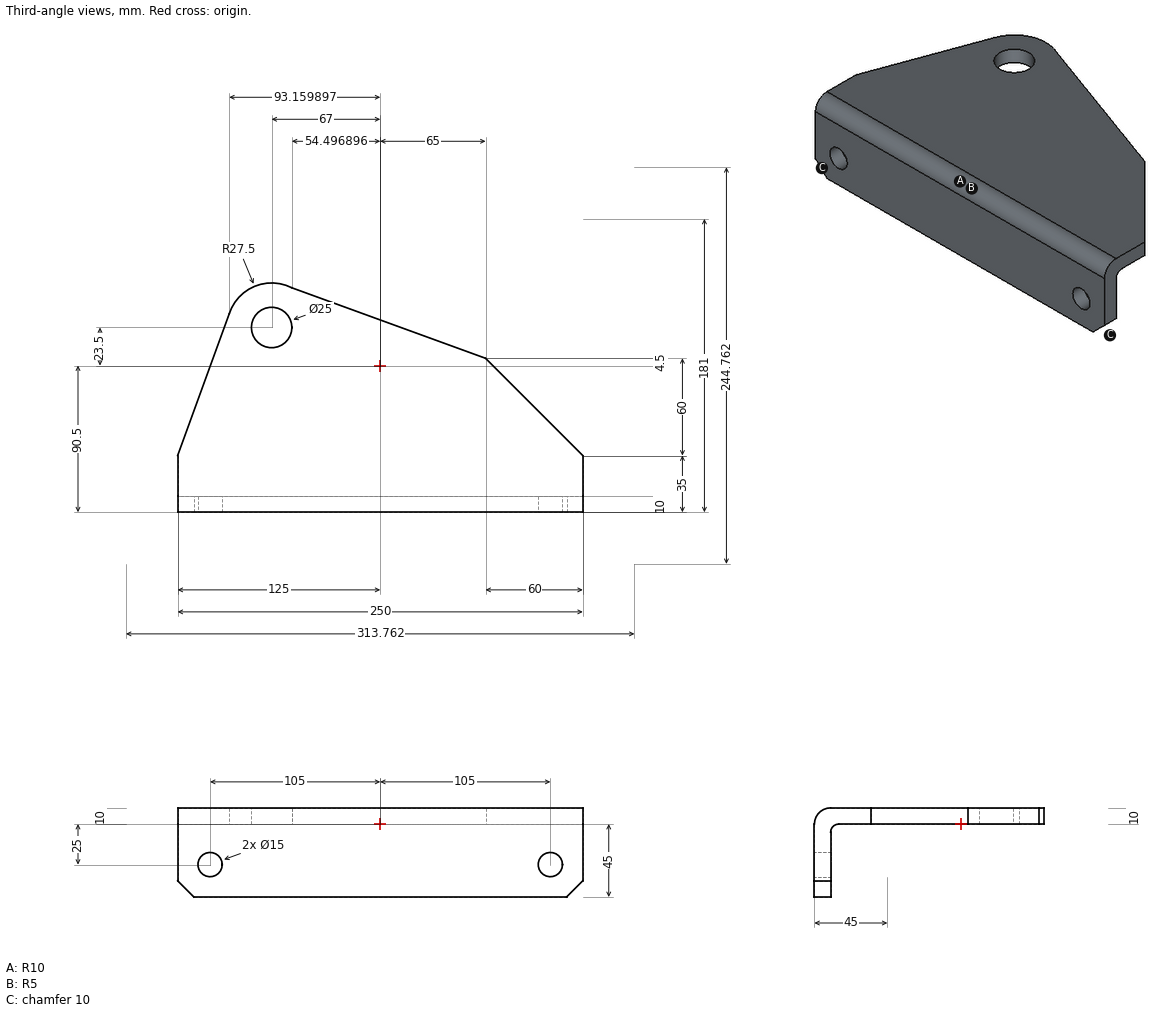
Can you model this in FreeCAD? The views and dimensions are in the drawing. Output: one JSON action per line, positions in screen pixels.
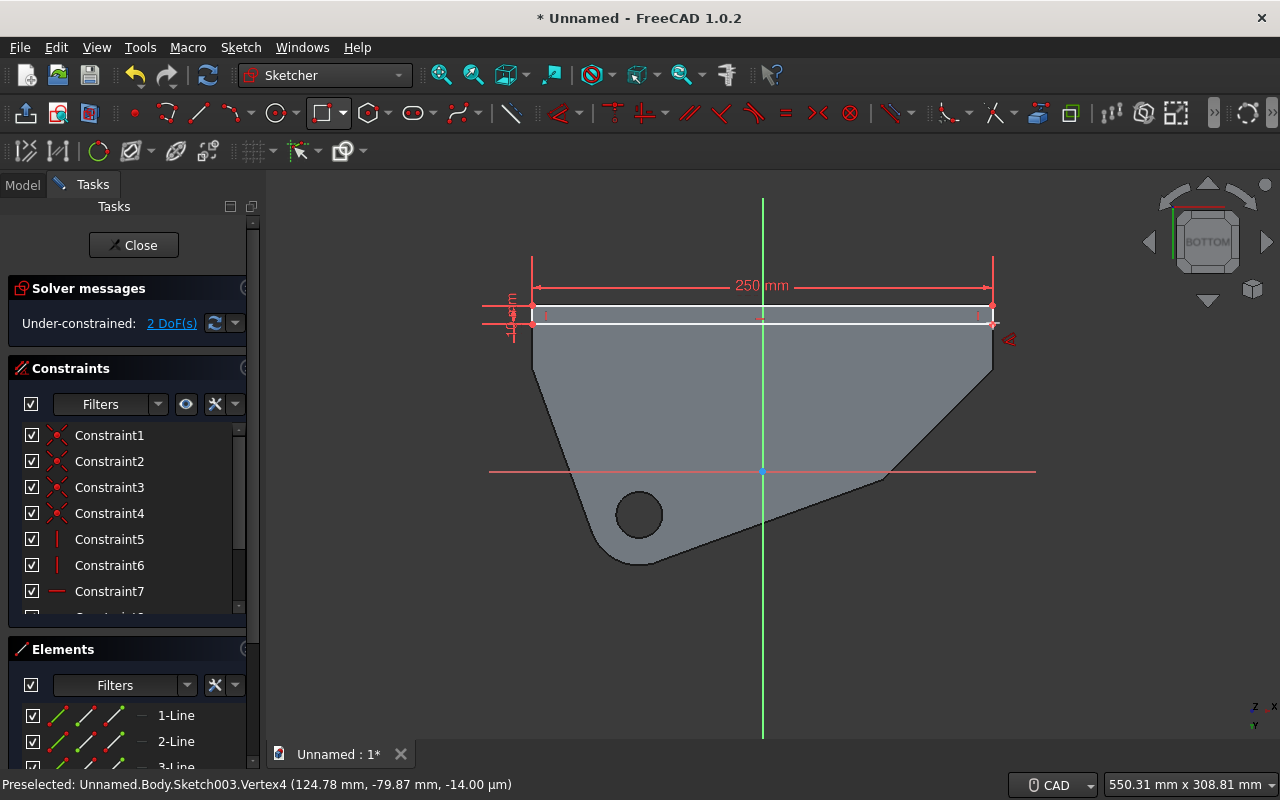
{"action": "left_click", "coordinate": [532, 306]}
{"action": "left_click", "coordinate": [647, 506]}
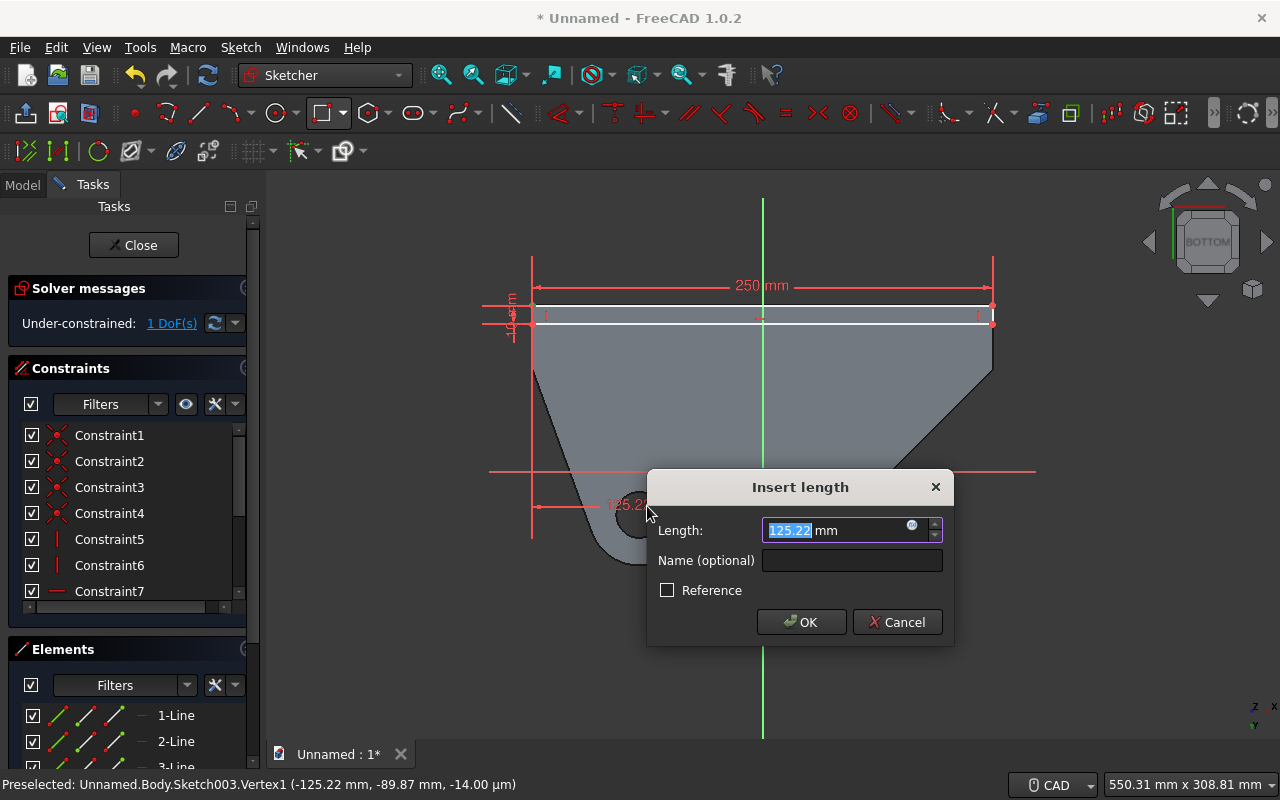
{"action": "type", "text": "125"}
{"action": "key", "text": "Return"}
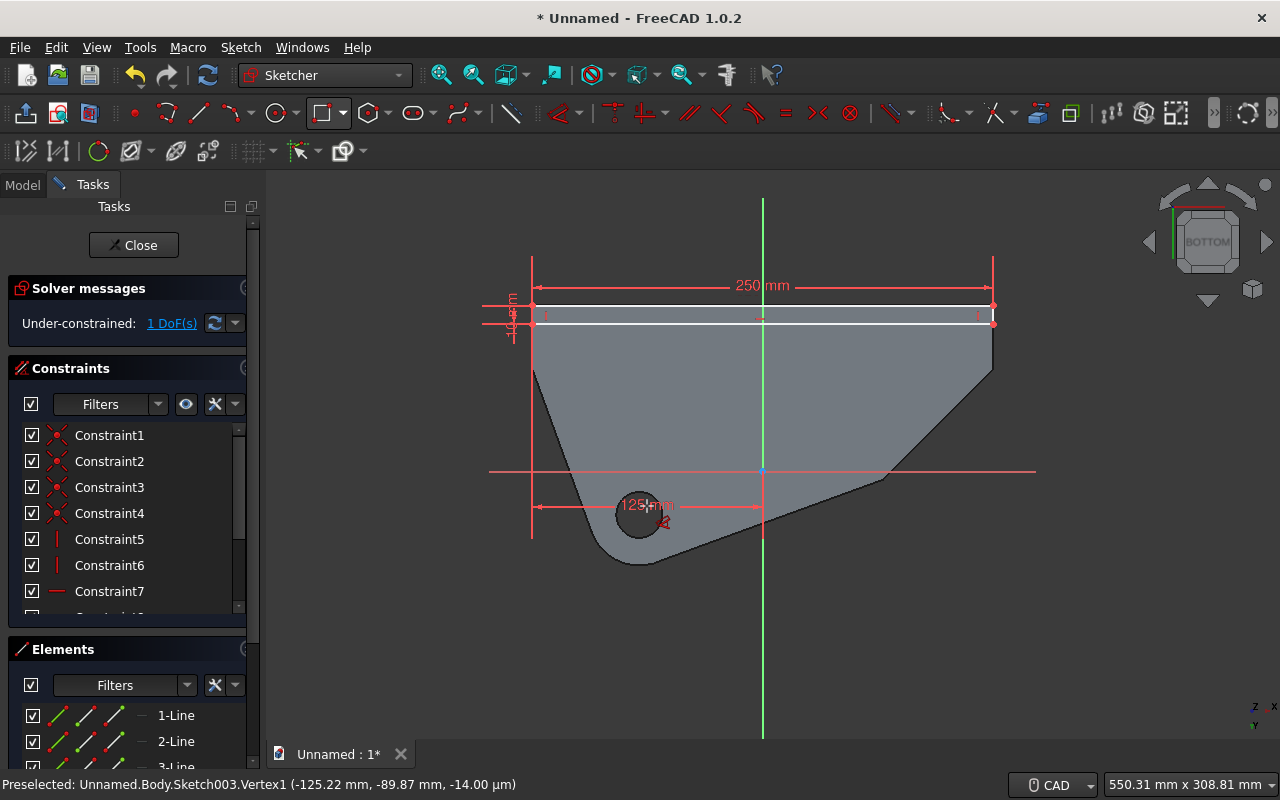
{"action": "left_click", "coordinate": [532, 306]}
{"action": "left_click", "coordinate": [498, 389]}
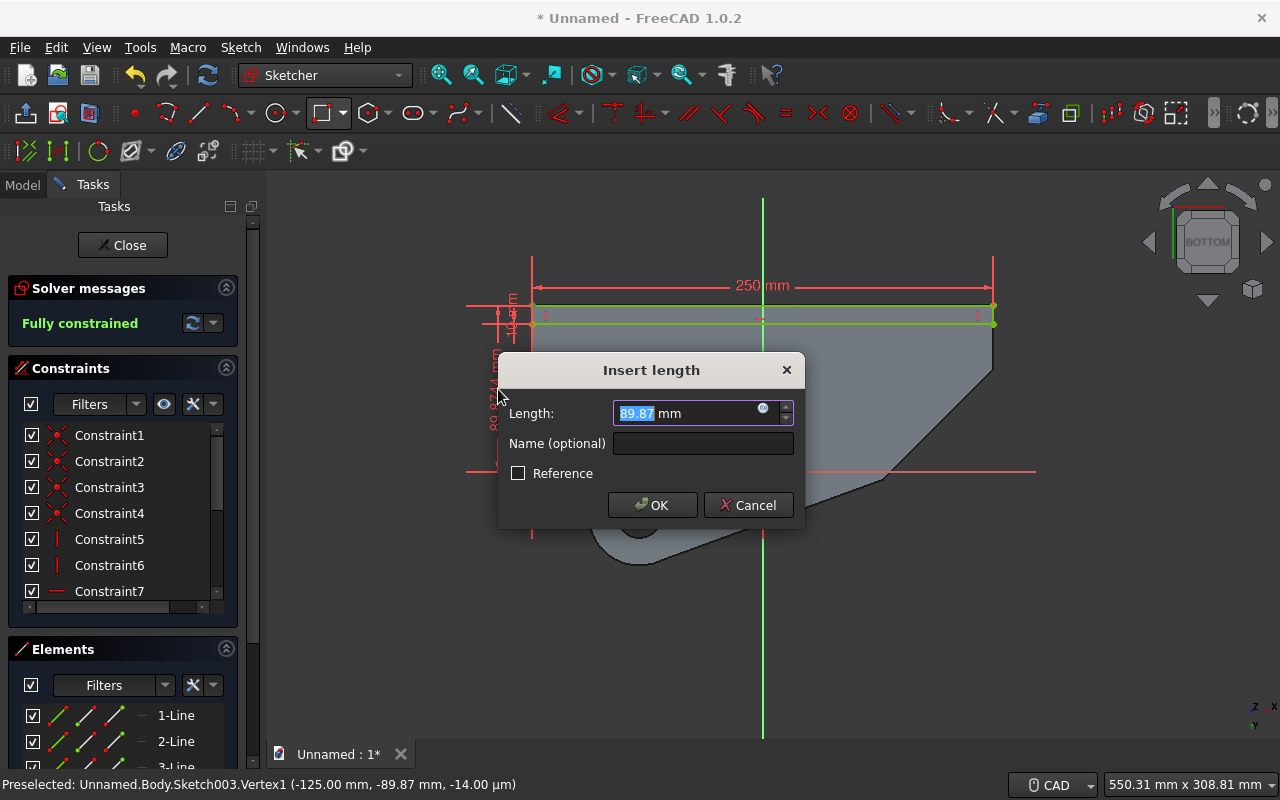
{"action": "type", "text": "90.5"}
{"action": "key", "text": "Return"}
{"action": "key", "text": "Escape"}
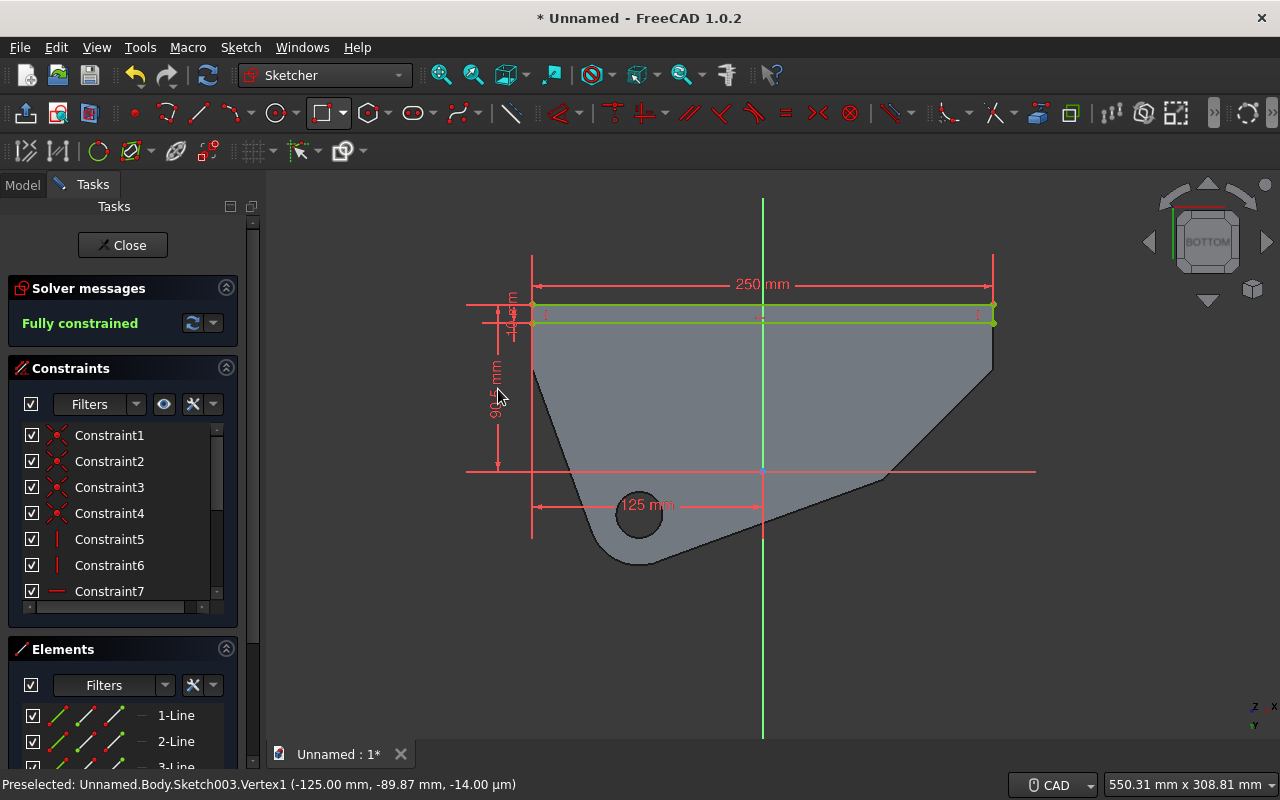
{"action": "left_click", "coordinate": [123, 245]}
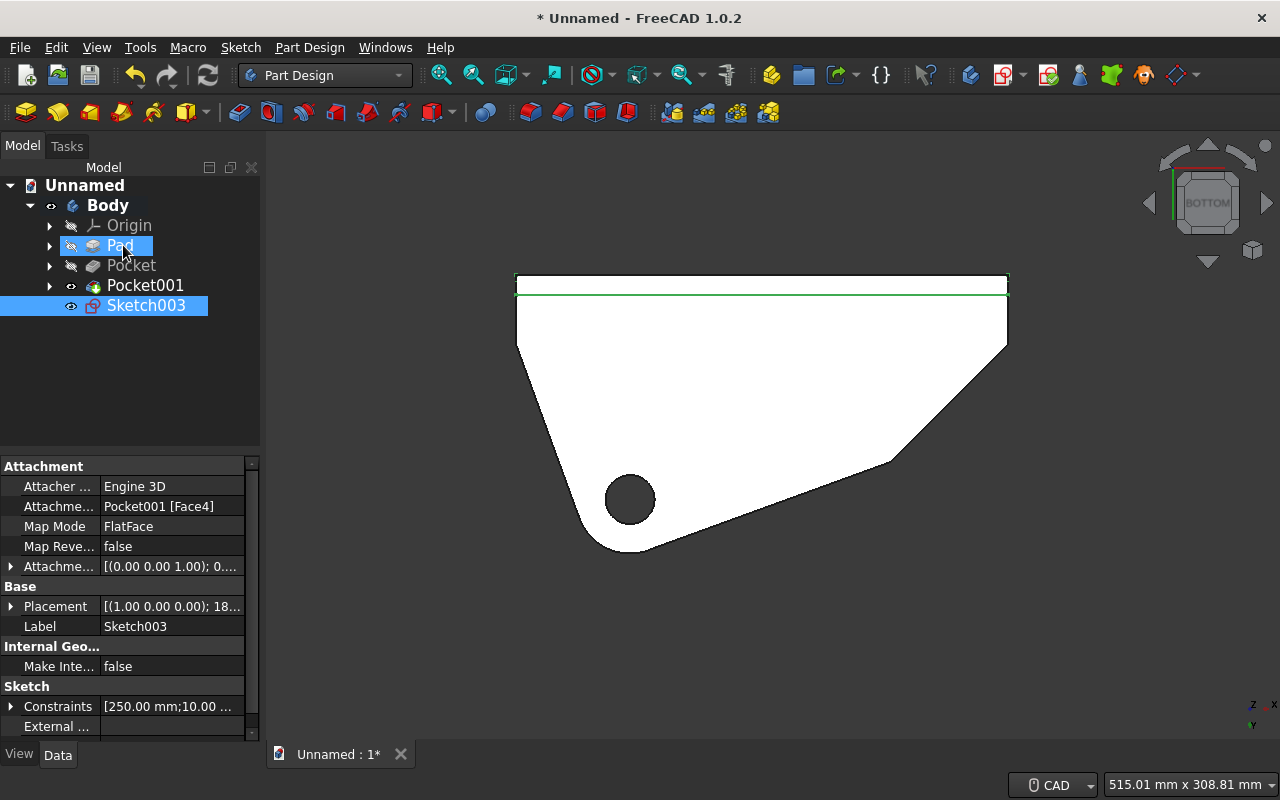
{"action": "left_click", "coordinate": [26, 112]}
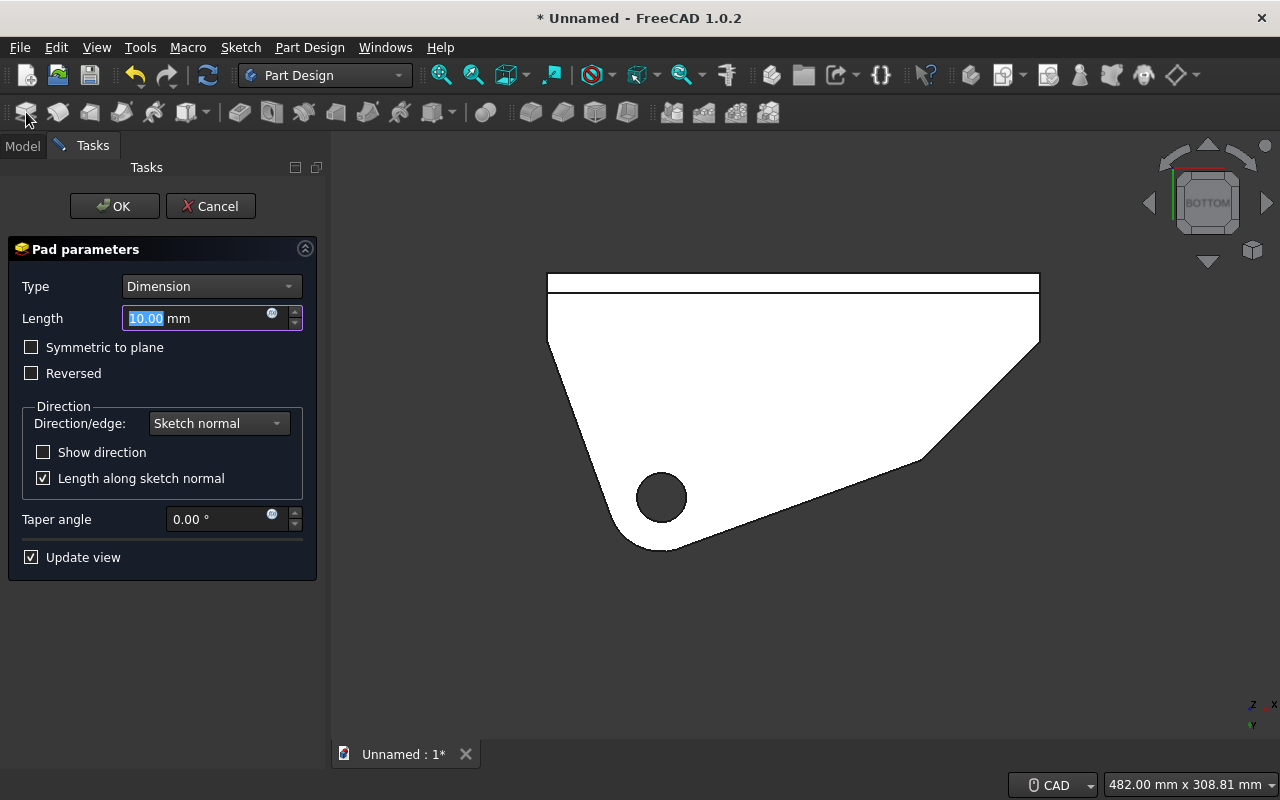
{"action": "type", "text": "45"}
{"action": "key", "text": "Tab"}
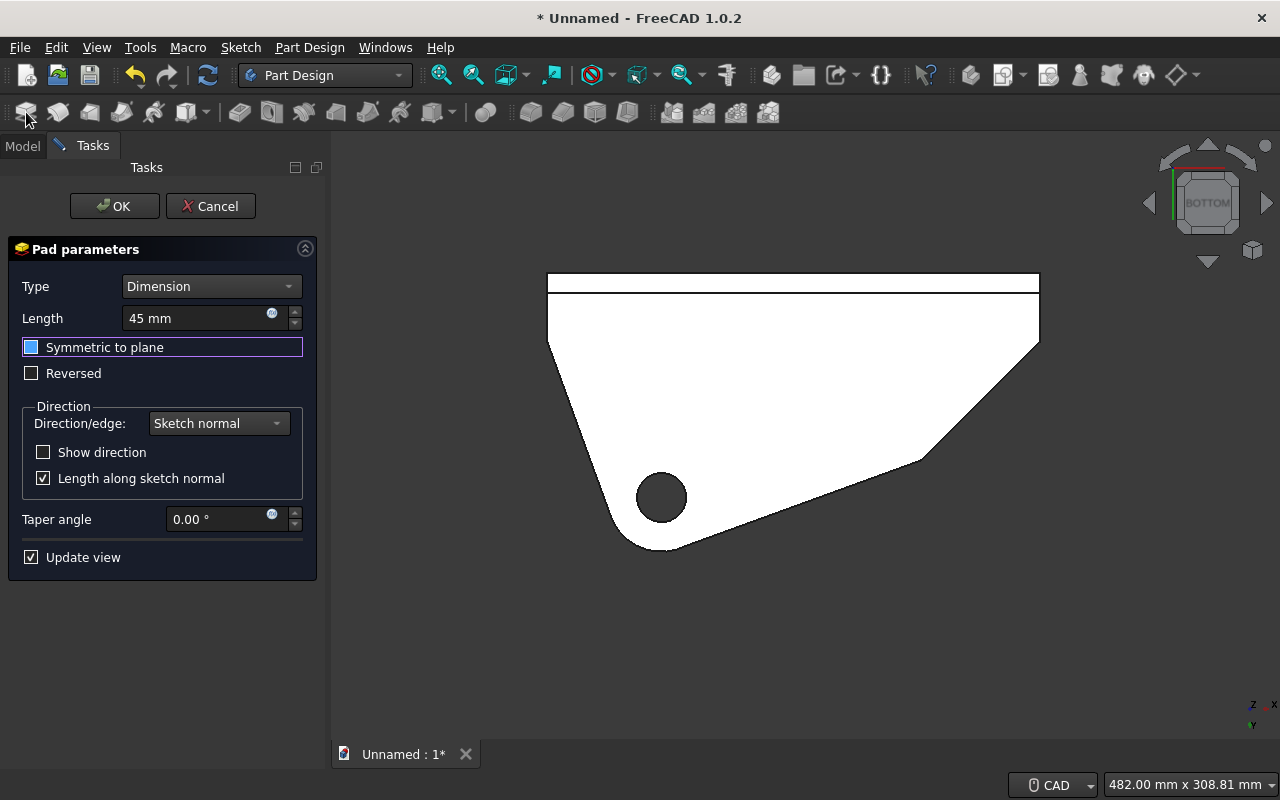
{"action": "left_click", "coordinate": [115, 206]}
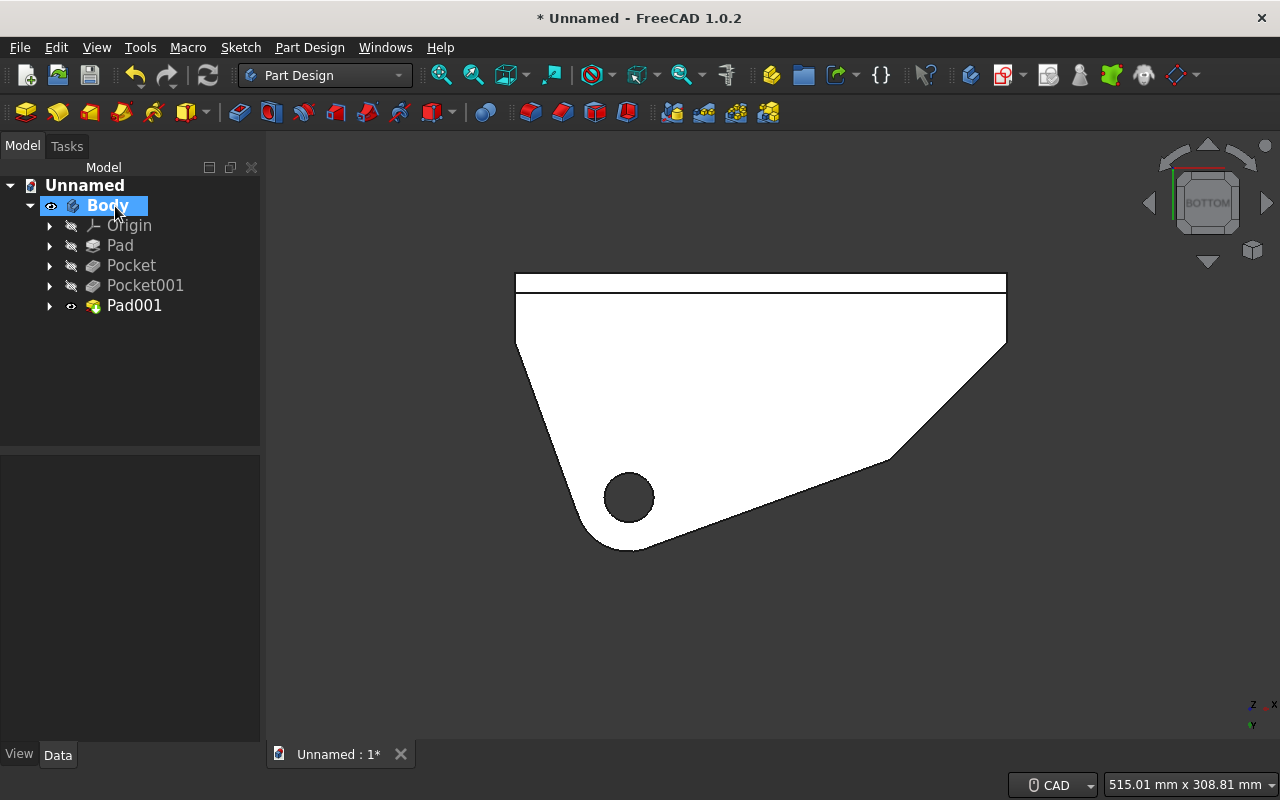
{"action": "key", "text": "0"}